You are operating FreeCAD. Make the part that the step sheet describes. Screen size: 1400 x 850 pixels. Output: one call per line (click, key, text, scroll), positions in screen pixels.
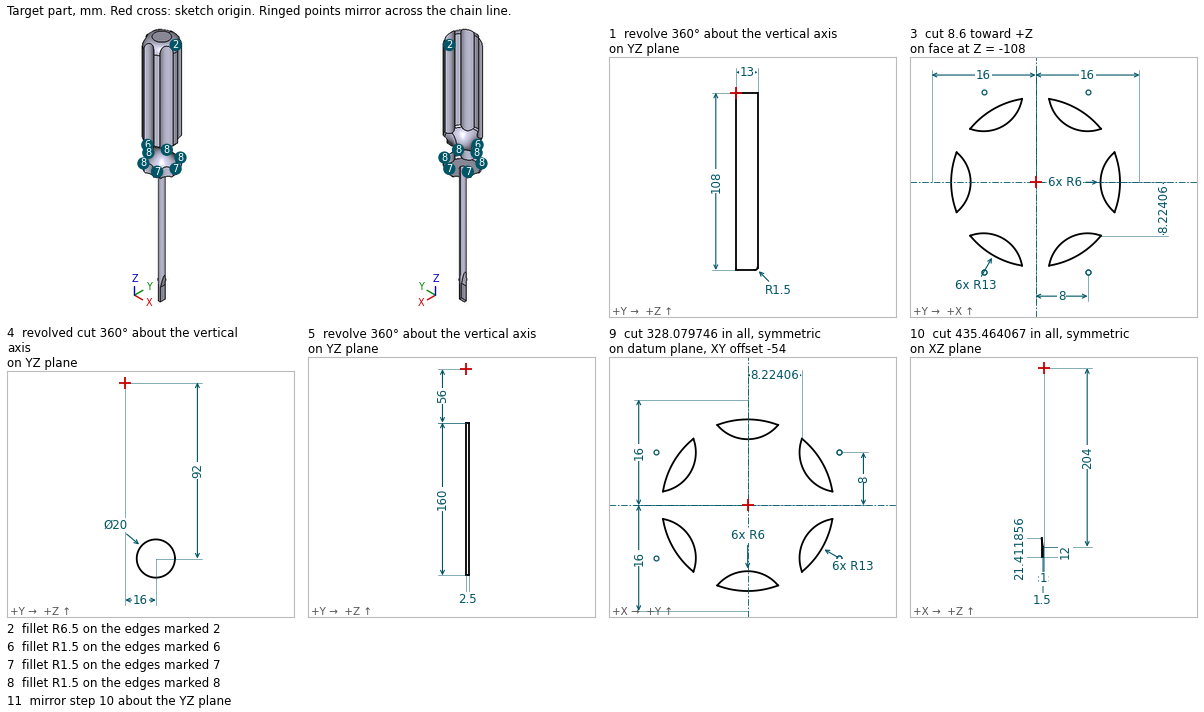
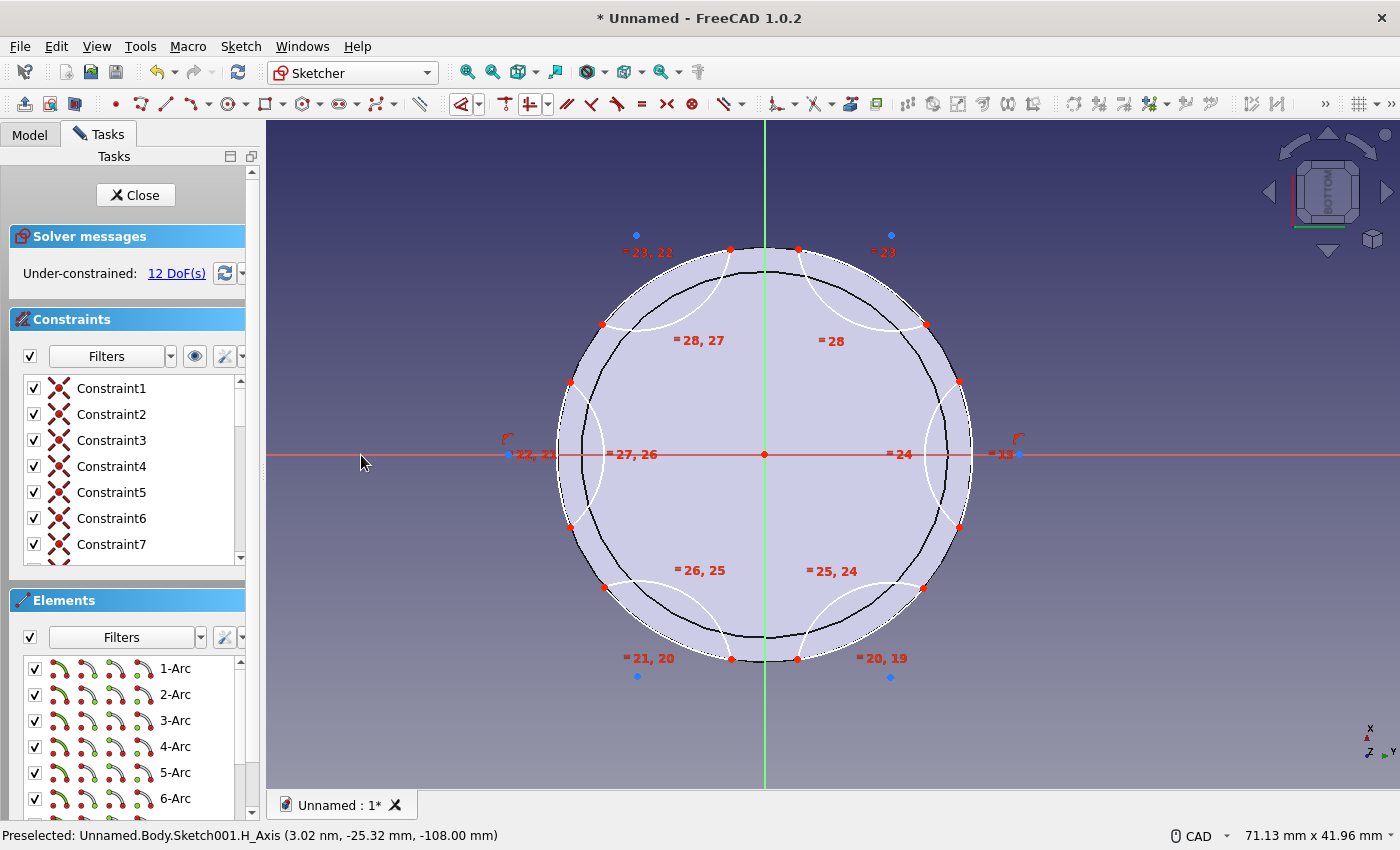
click(891, 678)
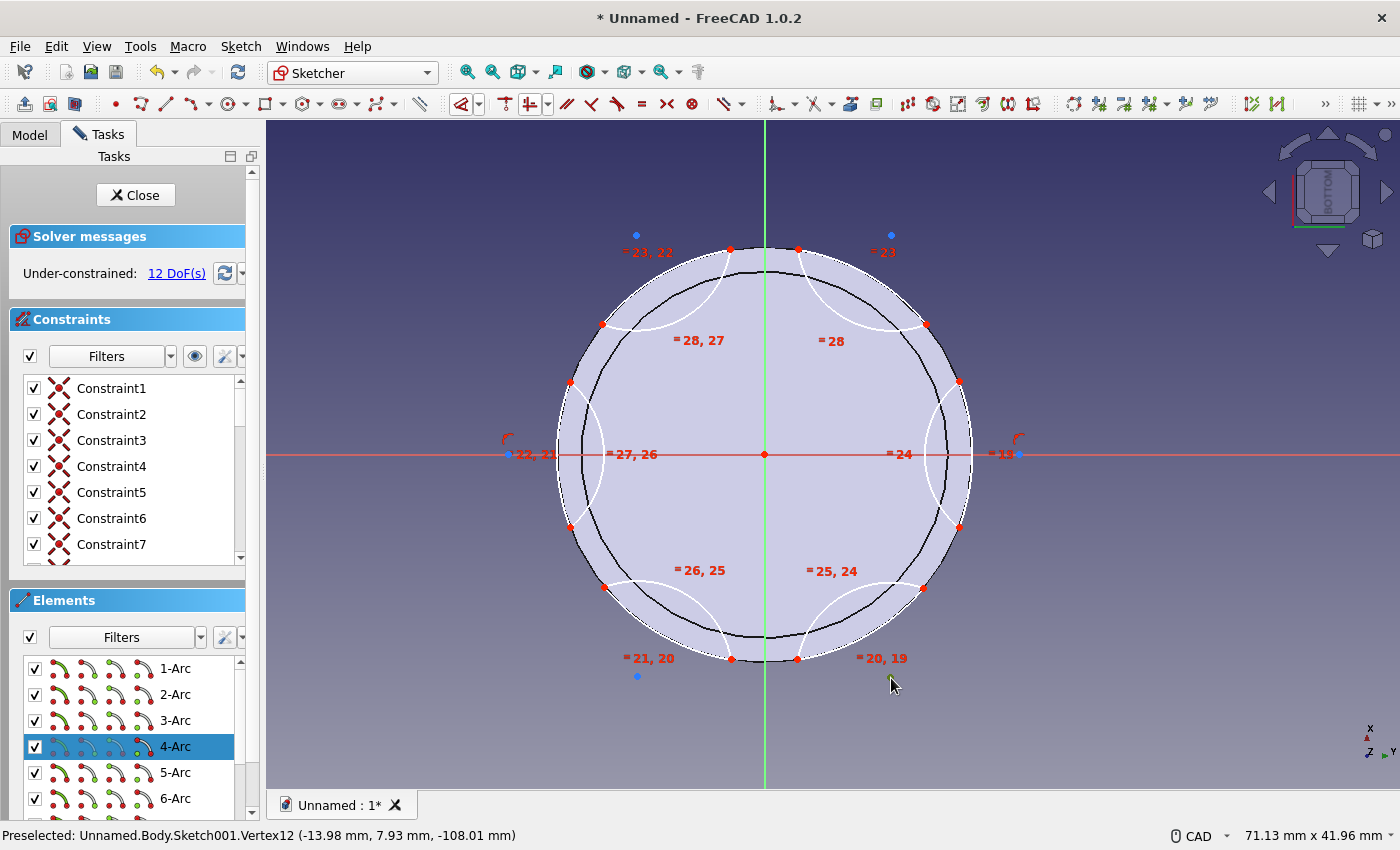
click(638, 676)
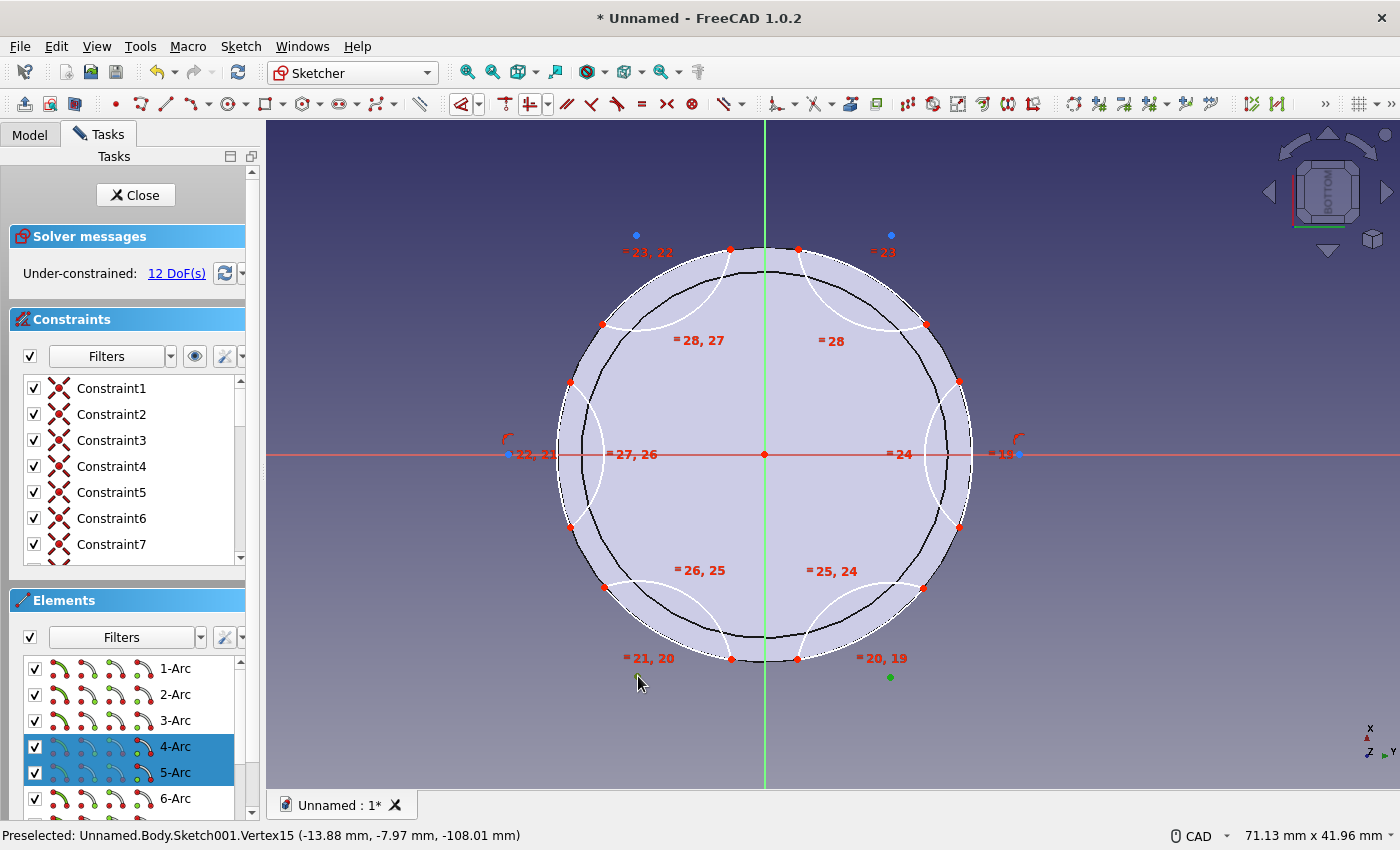
click(765, 717)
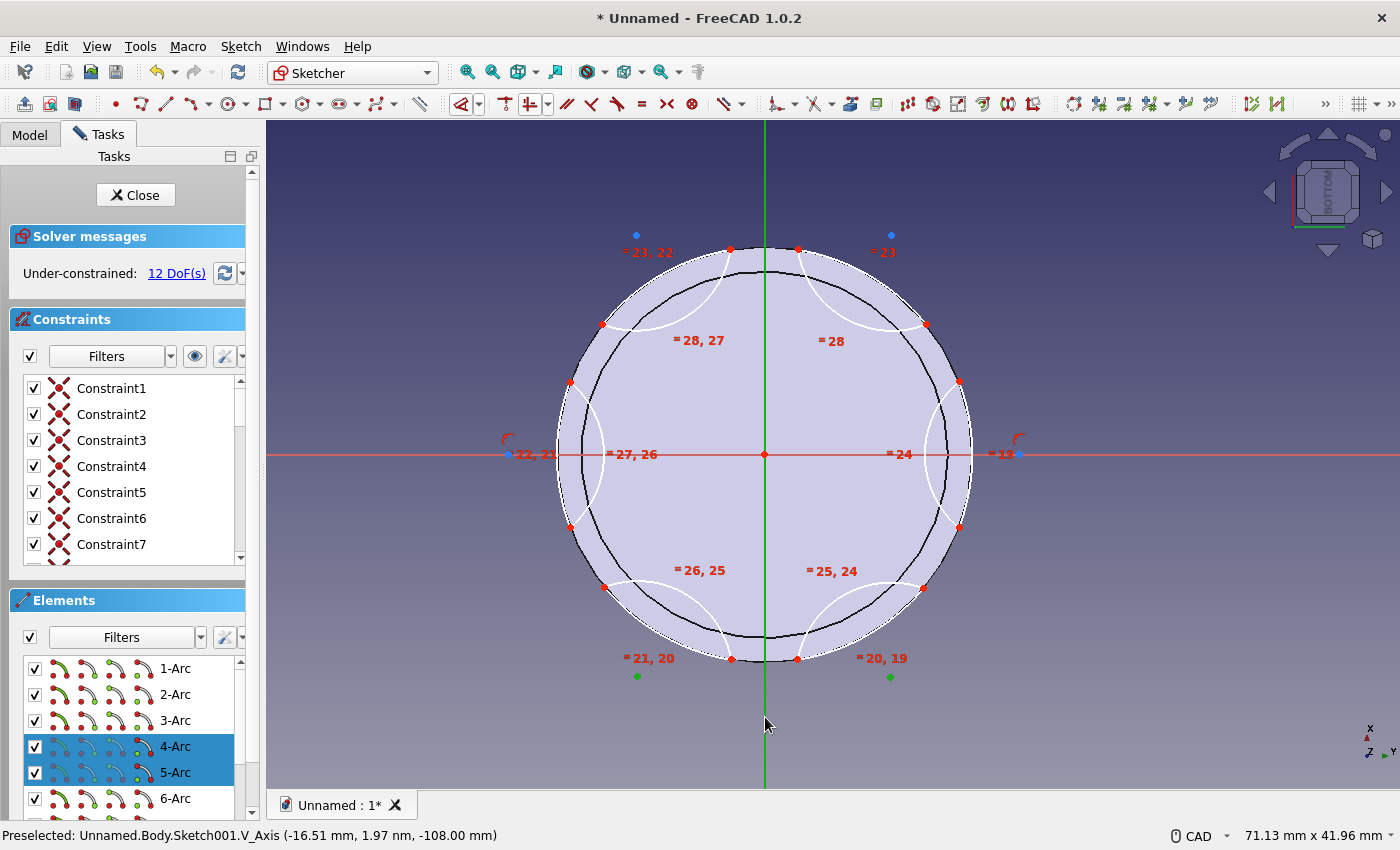
click(667, 104)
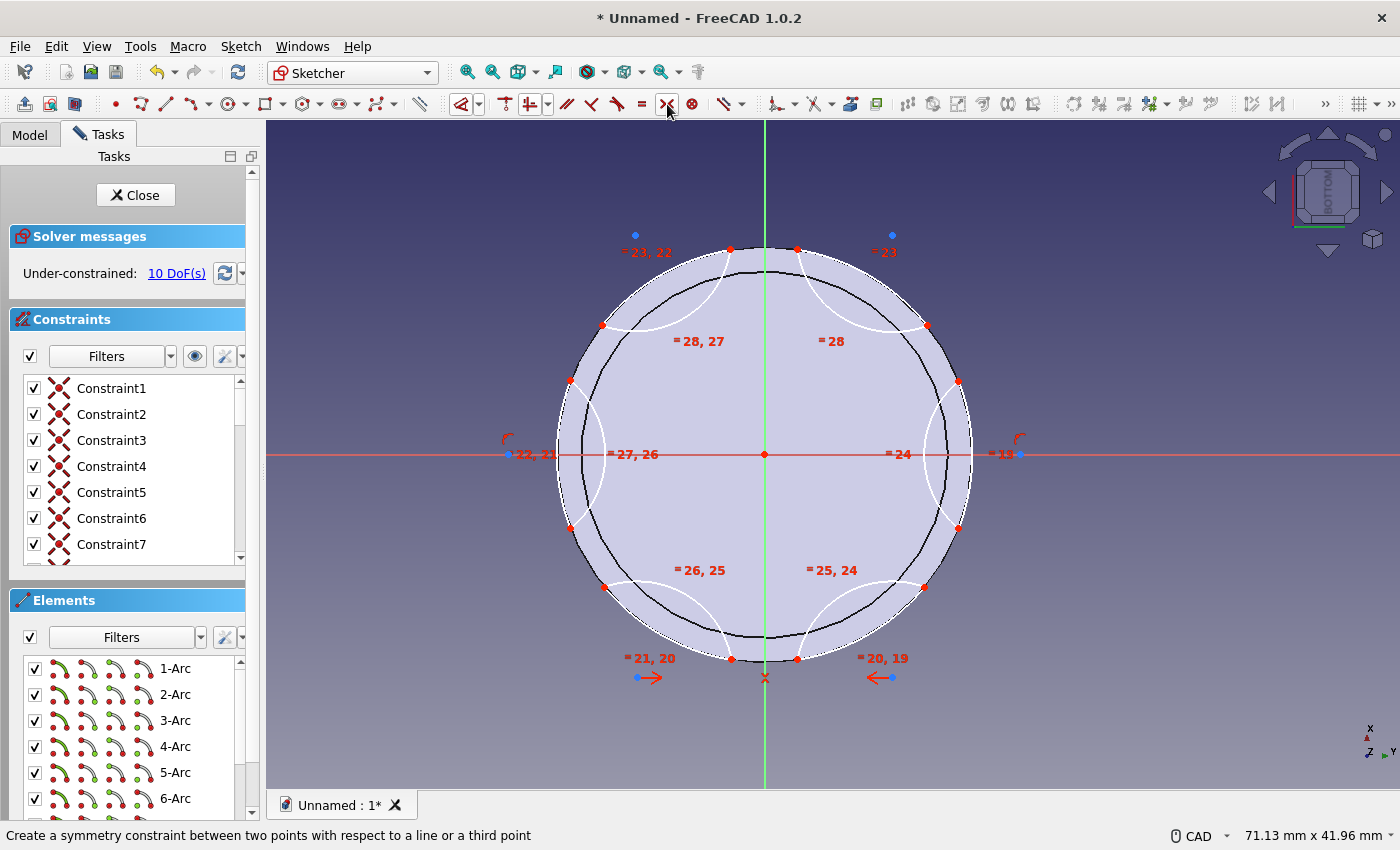
click(637, 678)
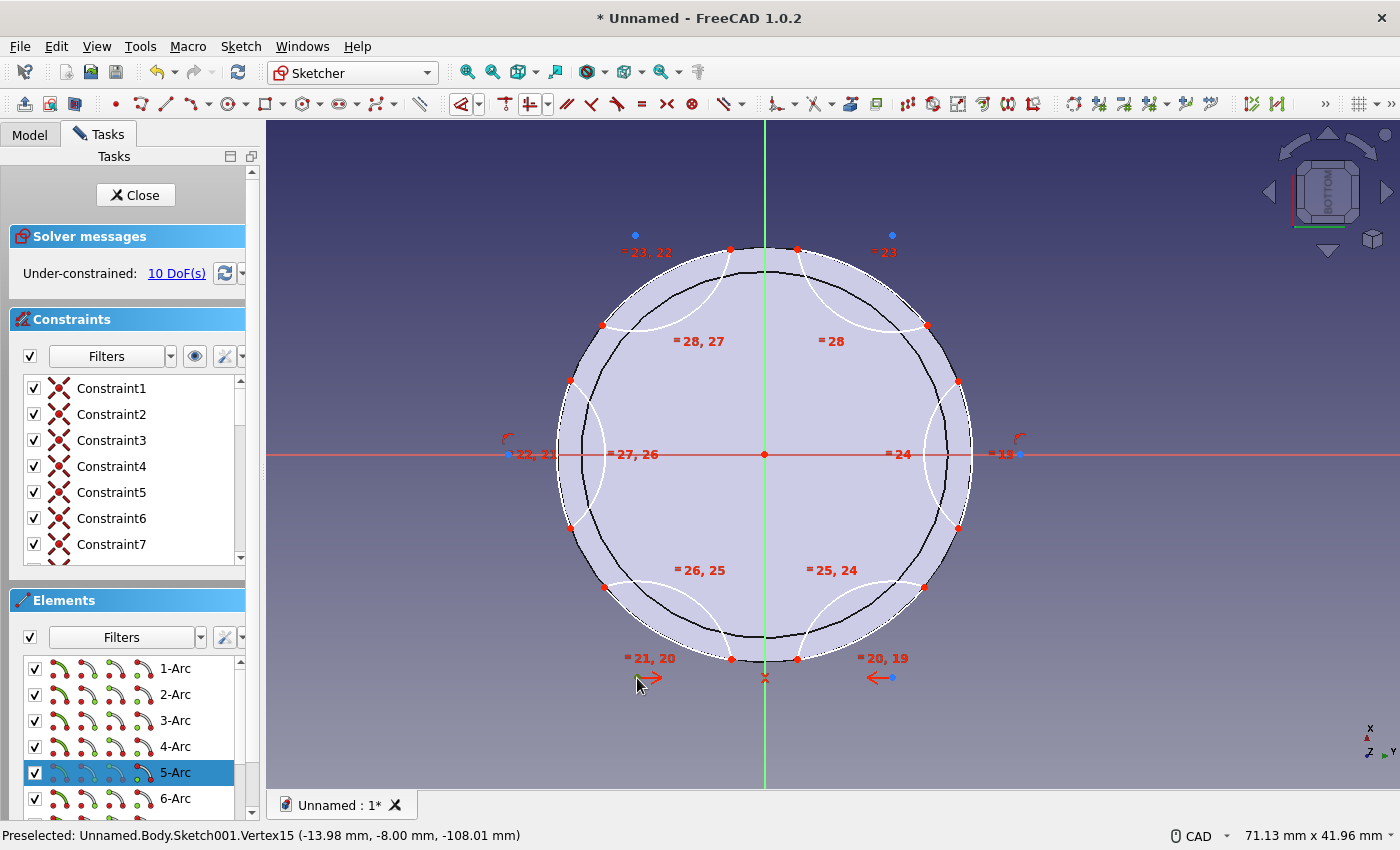
click(635, 235)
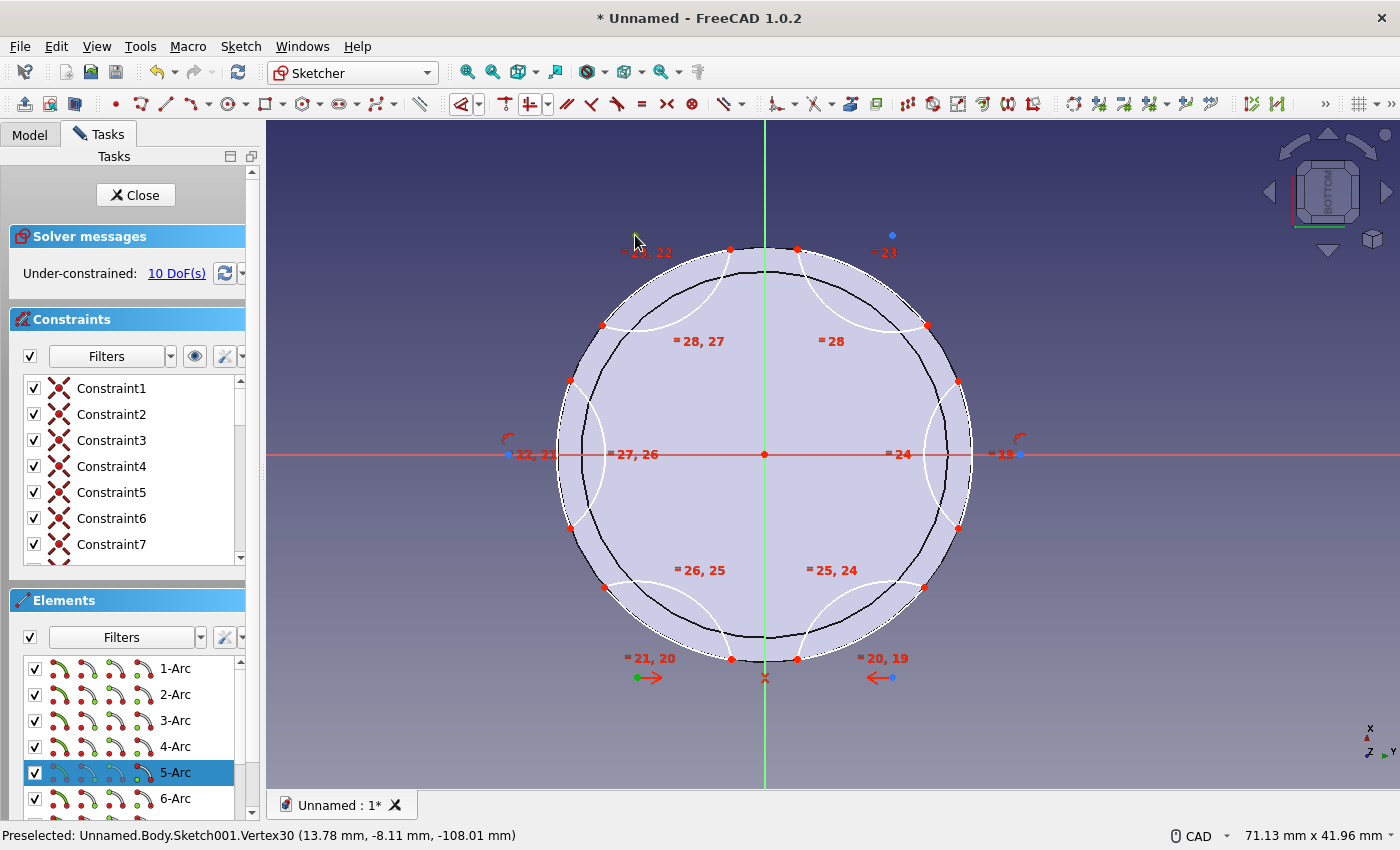
click(361, 455)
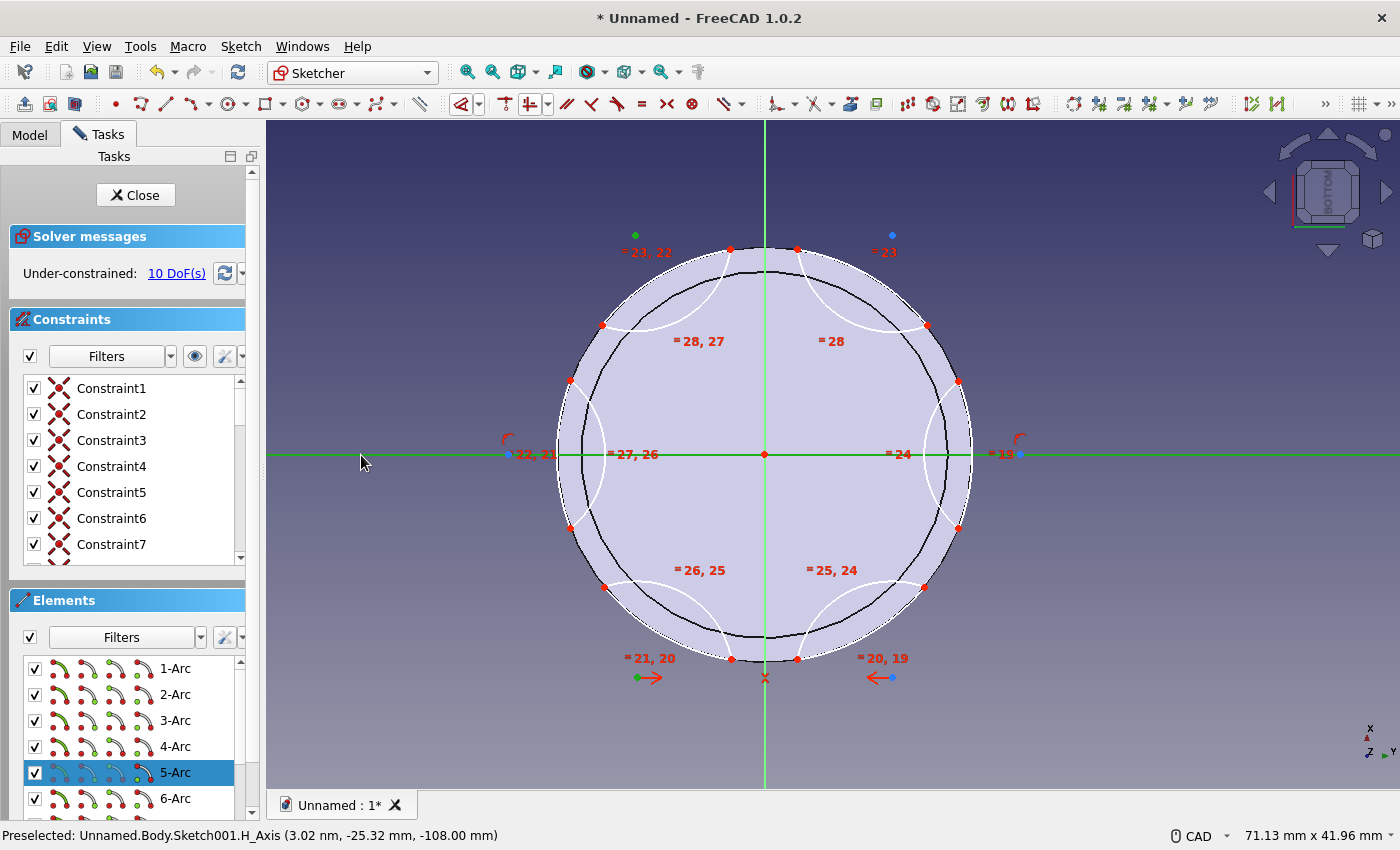
key(s)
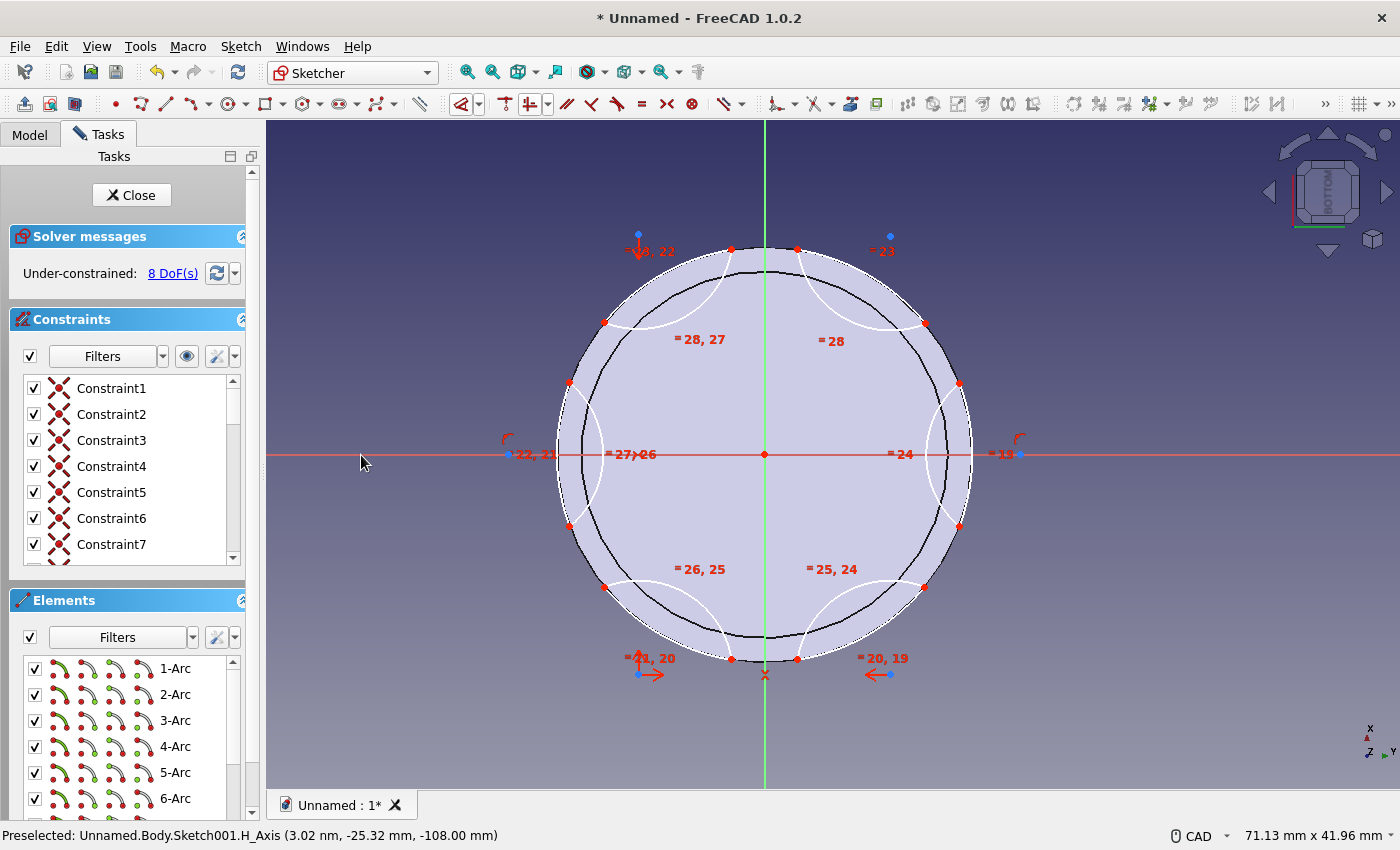
click(890, 675)